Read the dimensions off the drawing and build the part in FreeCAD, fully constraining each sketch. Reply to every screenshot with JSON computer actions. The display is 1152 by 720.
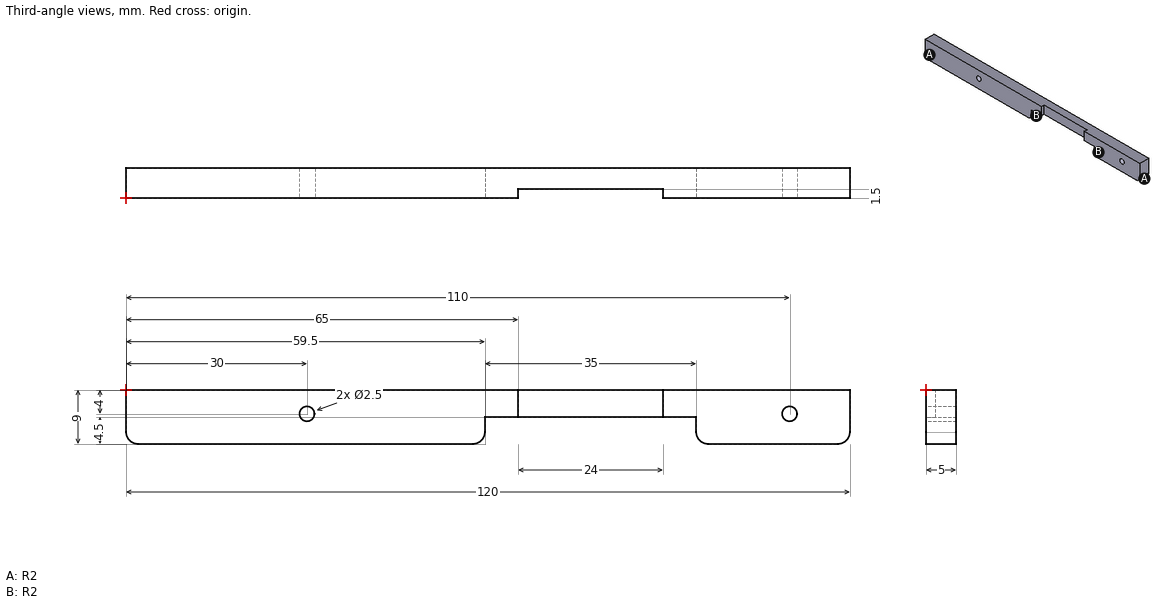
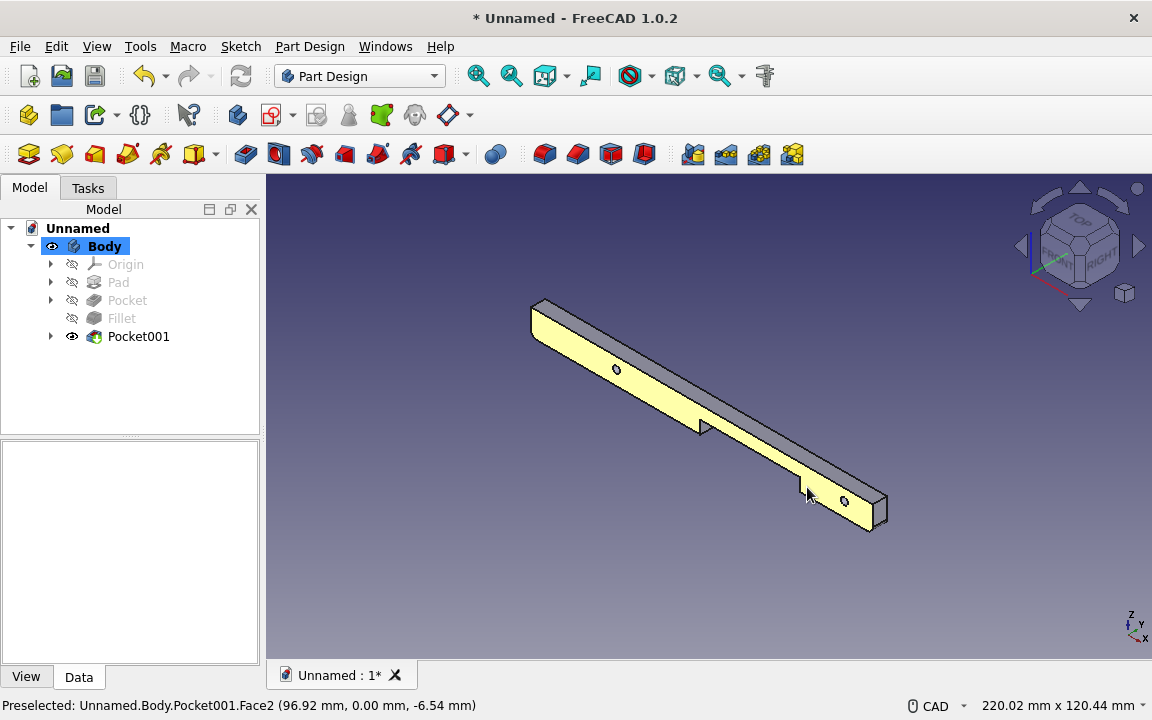
{"action": "scroll", "coordinate": [848, 415], "scroll_direction": "up", "scroll_amount": 4}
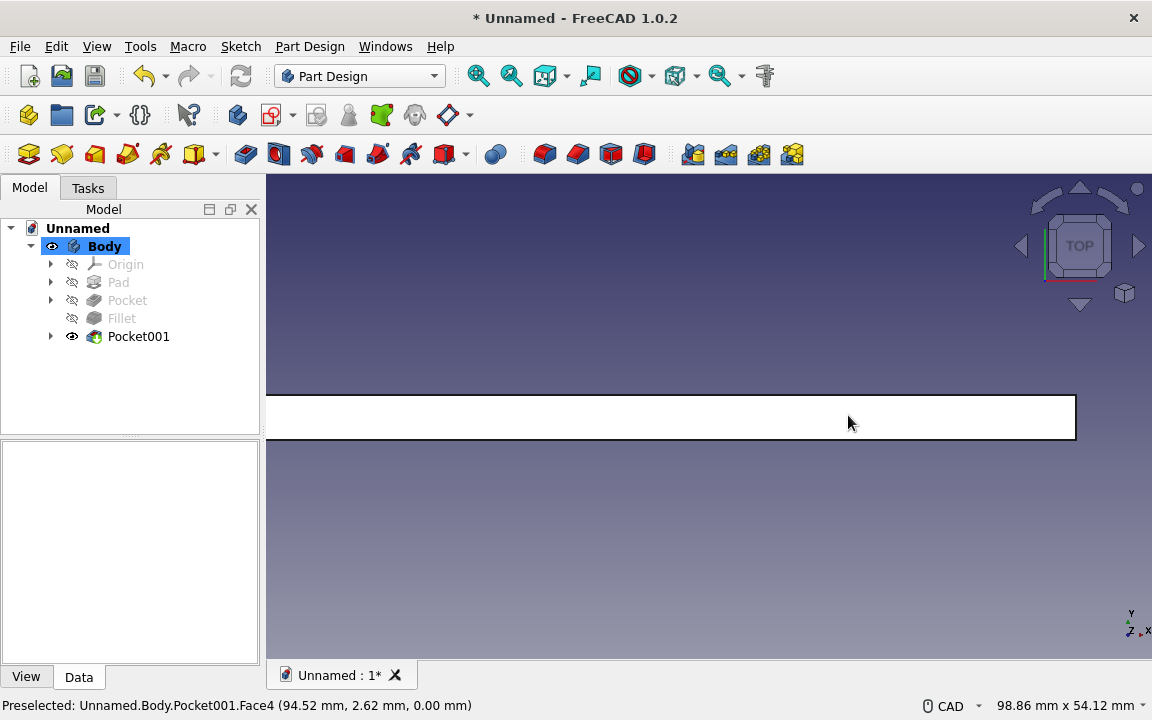
{"action": "key", "text": "v f"}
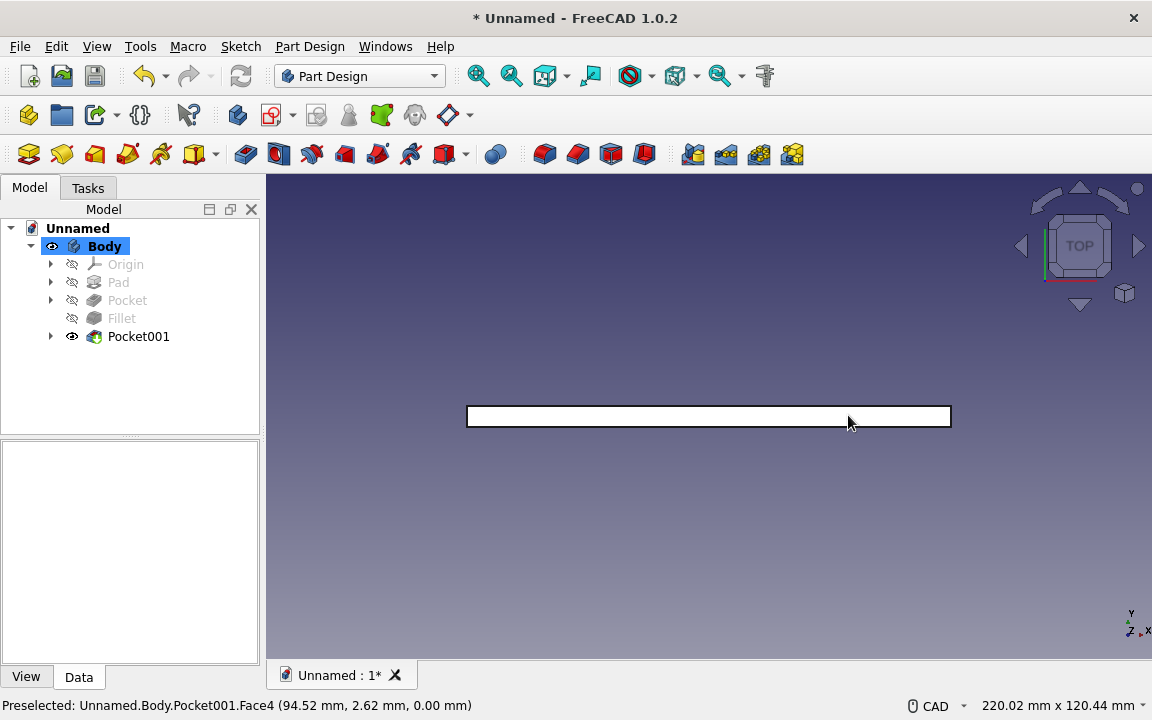
{"action": "key", "text": "1"}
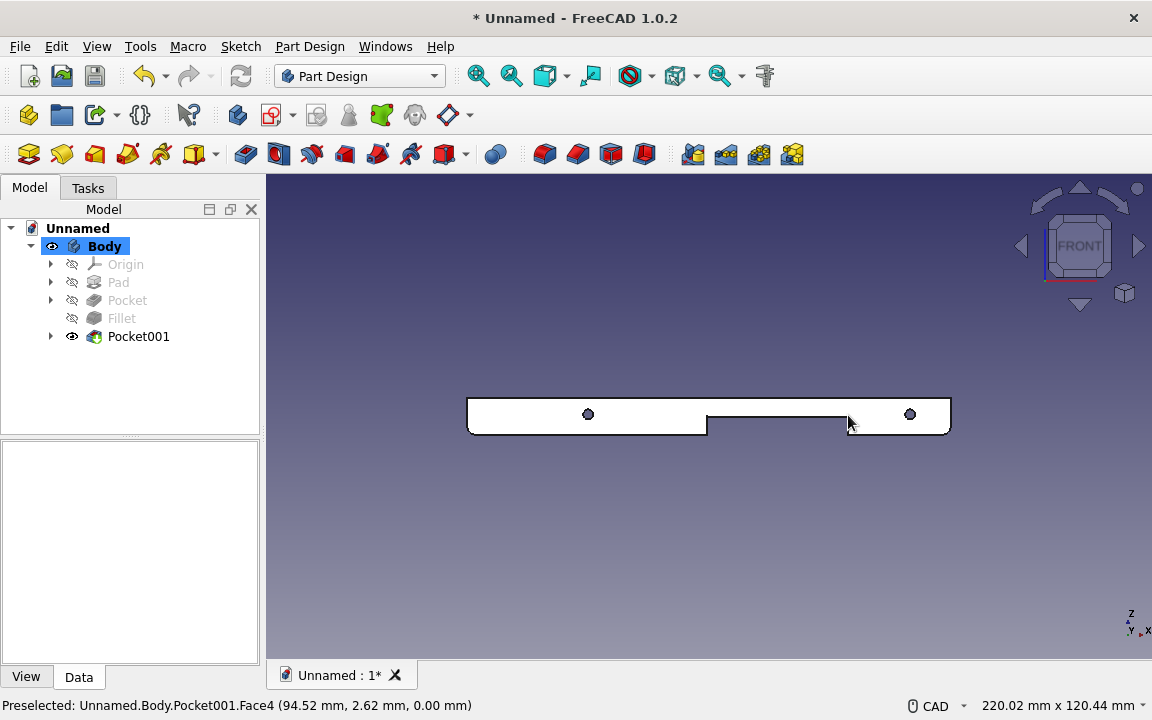
{"action": "scroll", "coordinate": [848, 434], "scroll_direction": "up", "scroll_amount": 4}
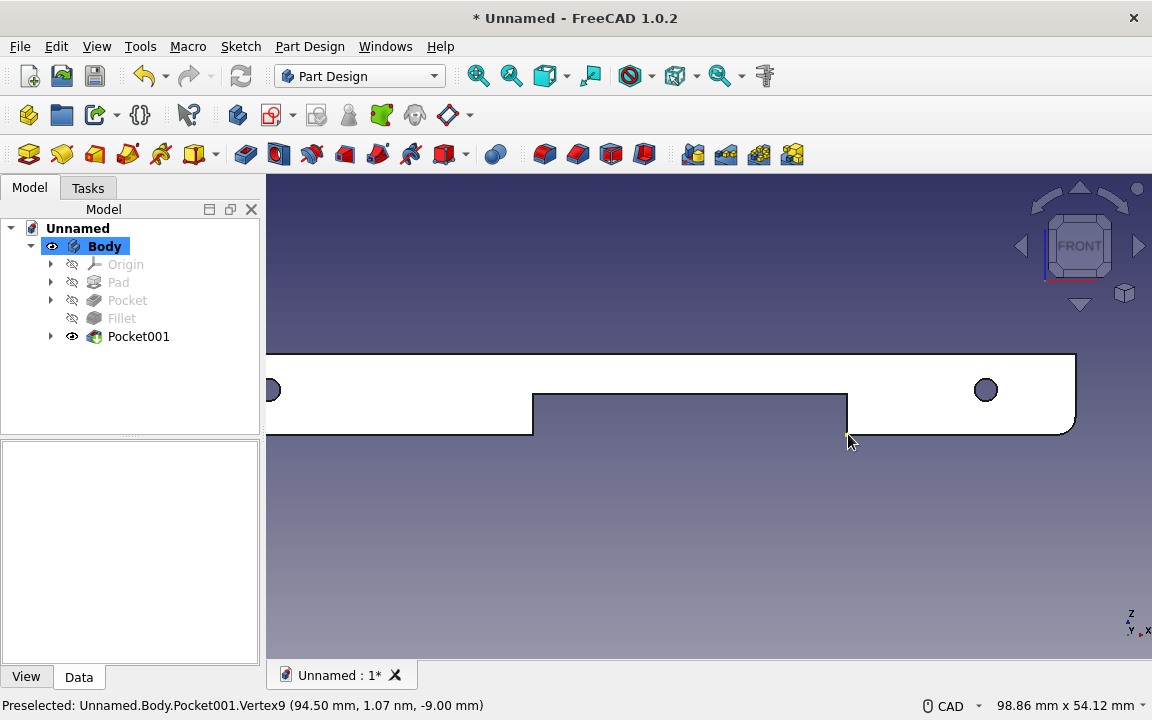
{"action": "key", "text": "v f"}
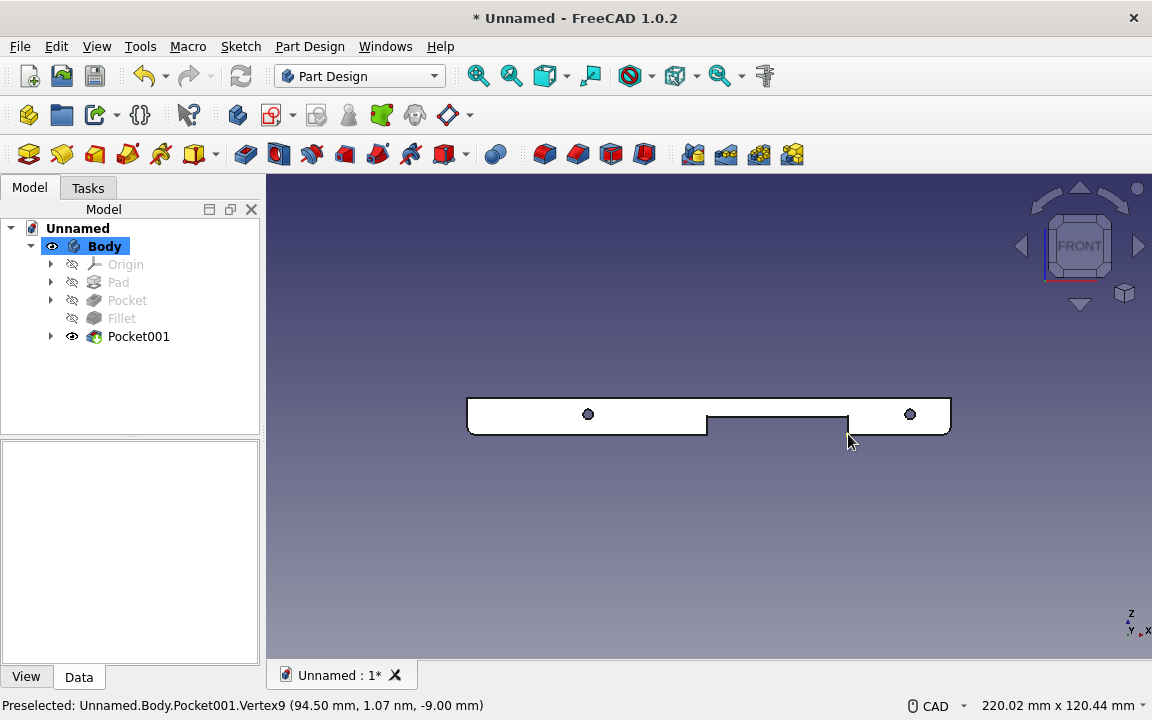
{"action": "key", "text": "3"}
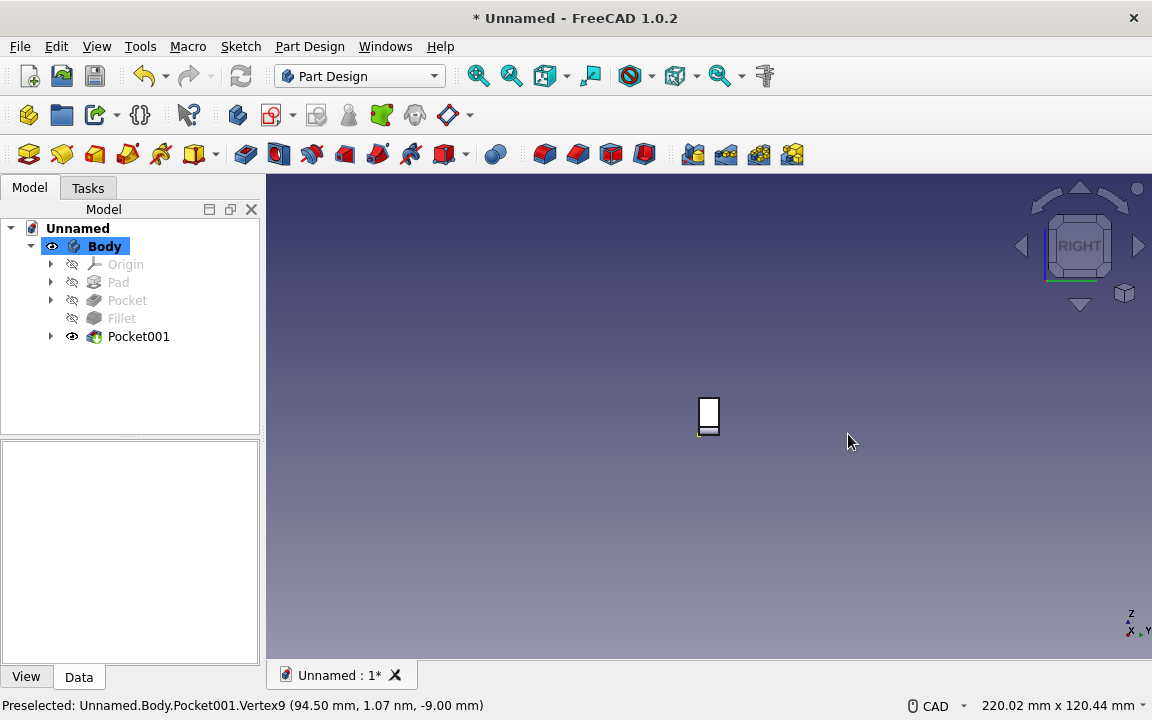
{"action": "key", "text": "v f"}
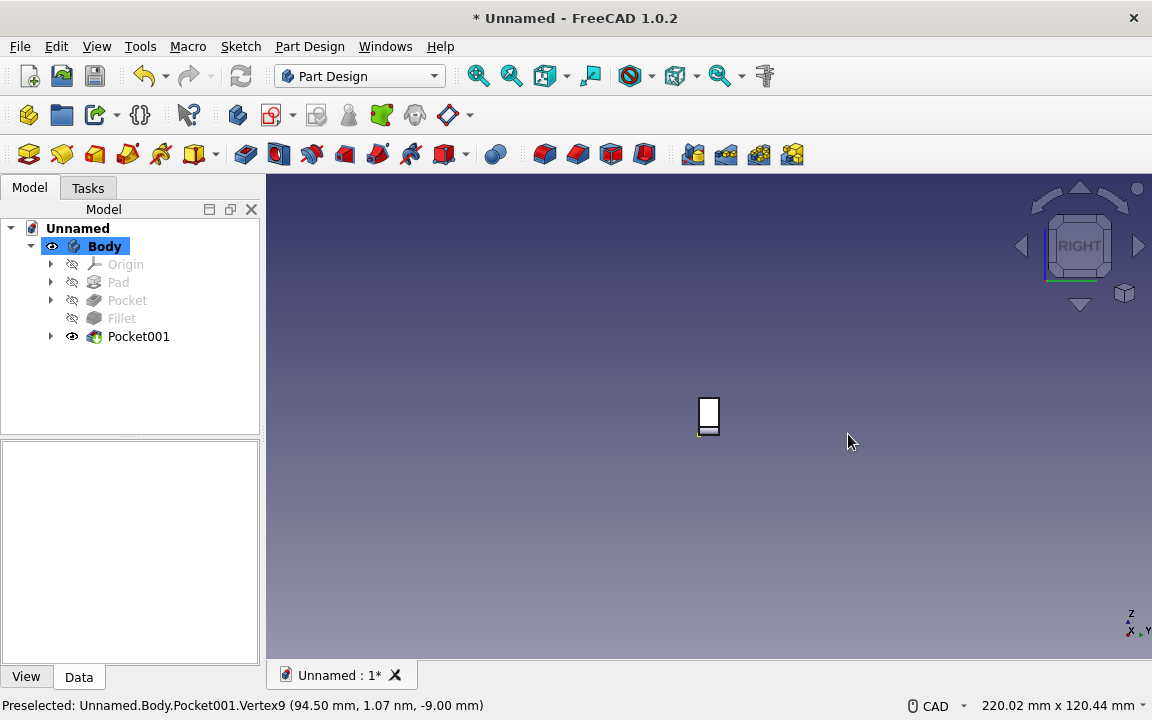
{"action": "scroll", "coordinate": [709, 434], "scroll_direction": "up", "scroll_amount": 4}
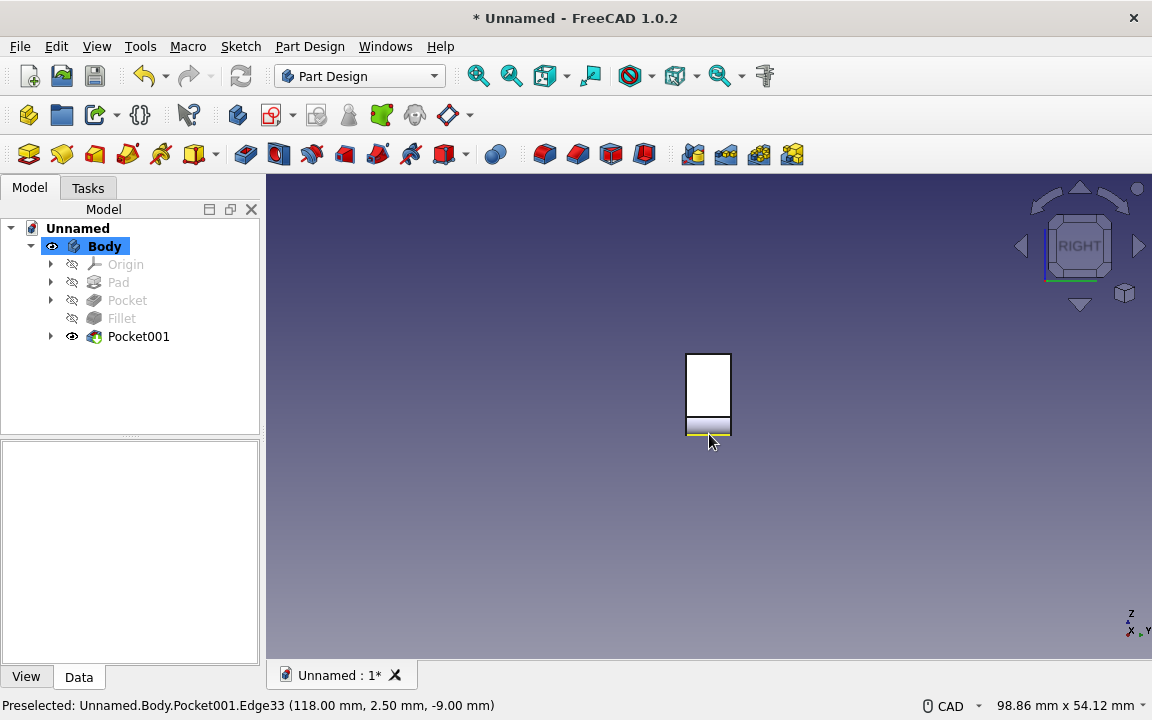
{"action": "key", "text": "v f"}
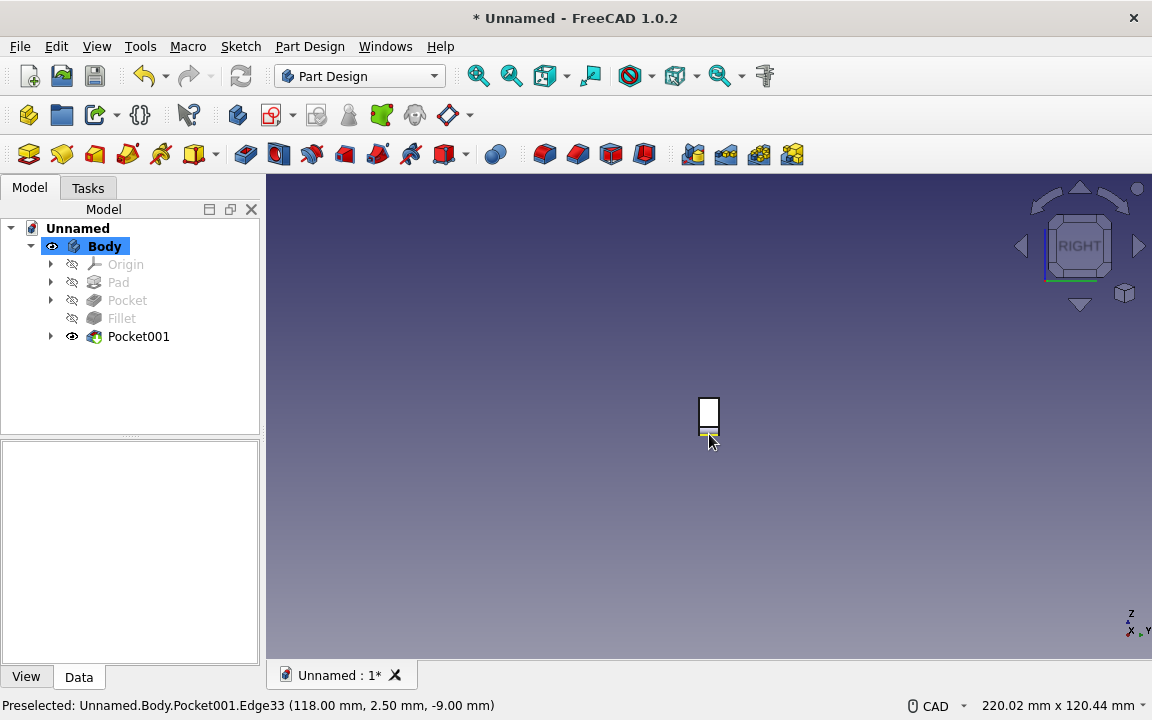
{"action": "key", "text": "5"}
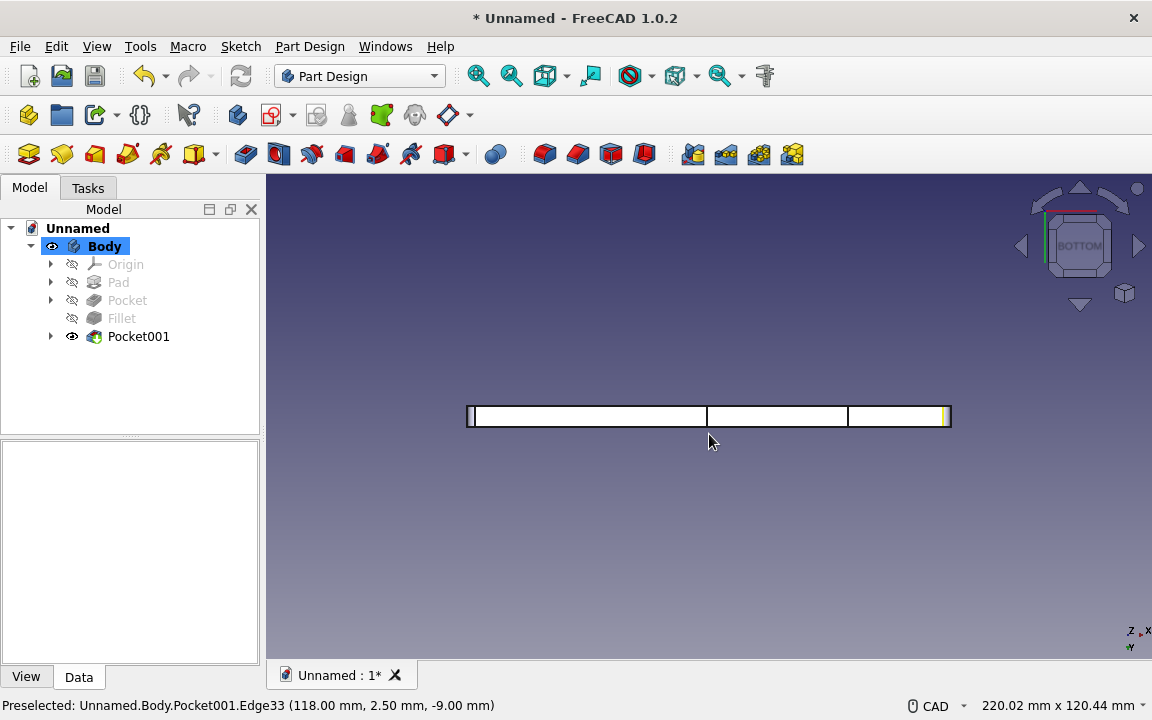
{"action": "left_click", "coordinate": [848, 415]}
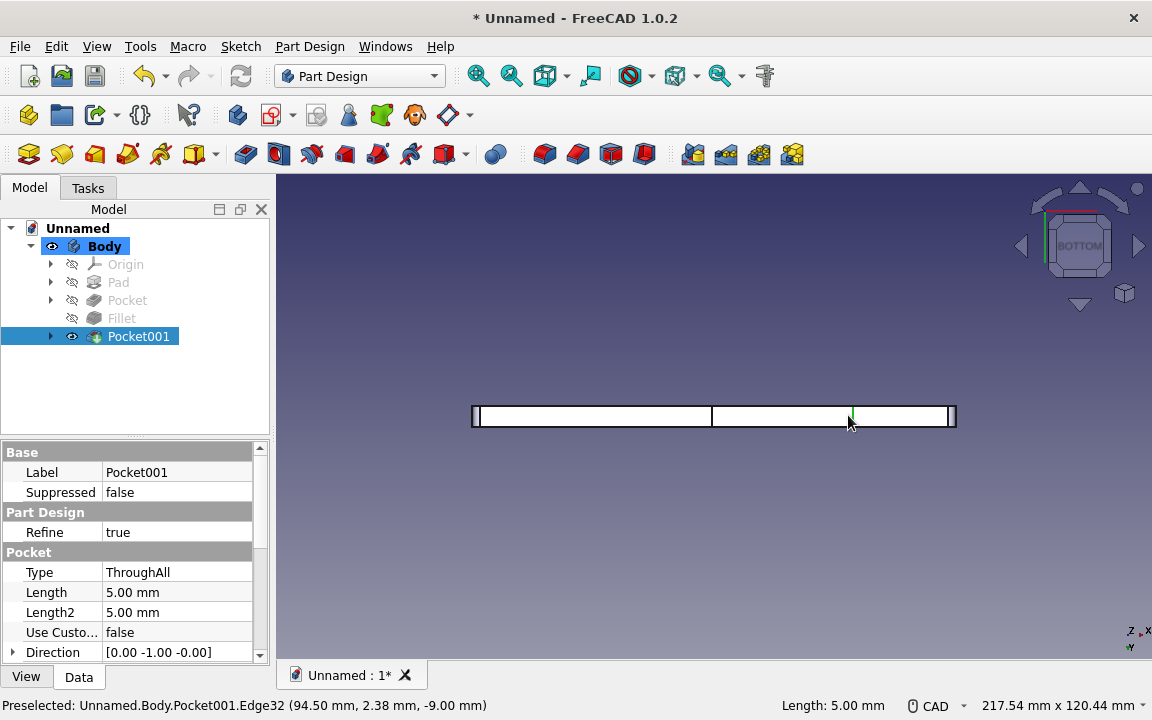
{"action": "left_click", "coordinate": [712, 415], "text": "ctrl"}